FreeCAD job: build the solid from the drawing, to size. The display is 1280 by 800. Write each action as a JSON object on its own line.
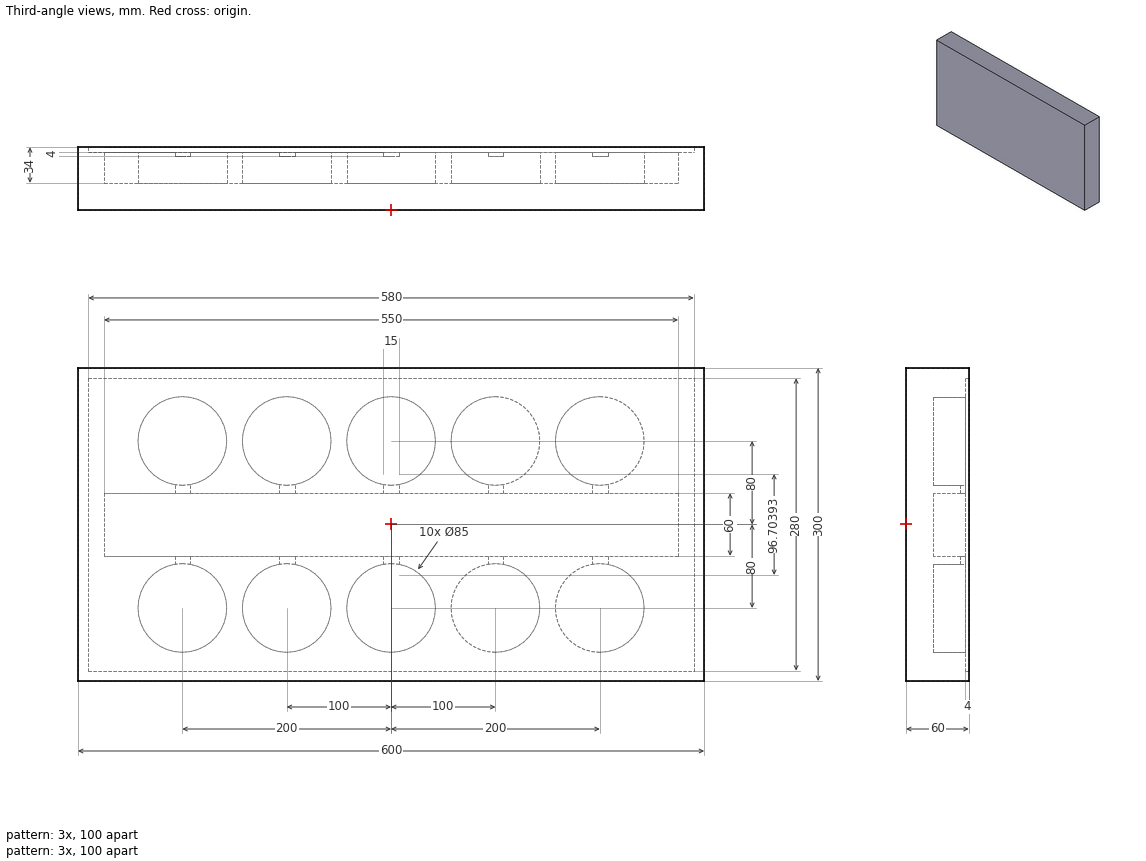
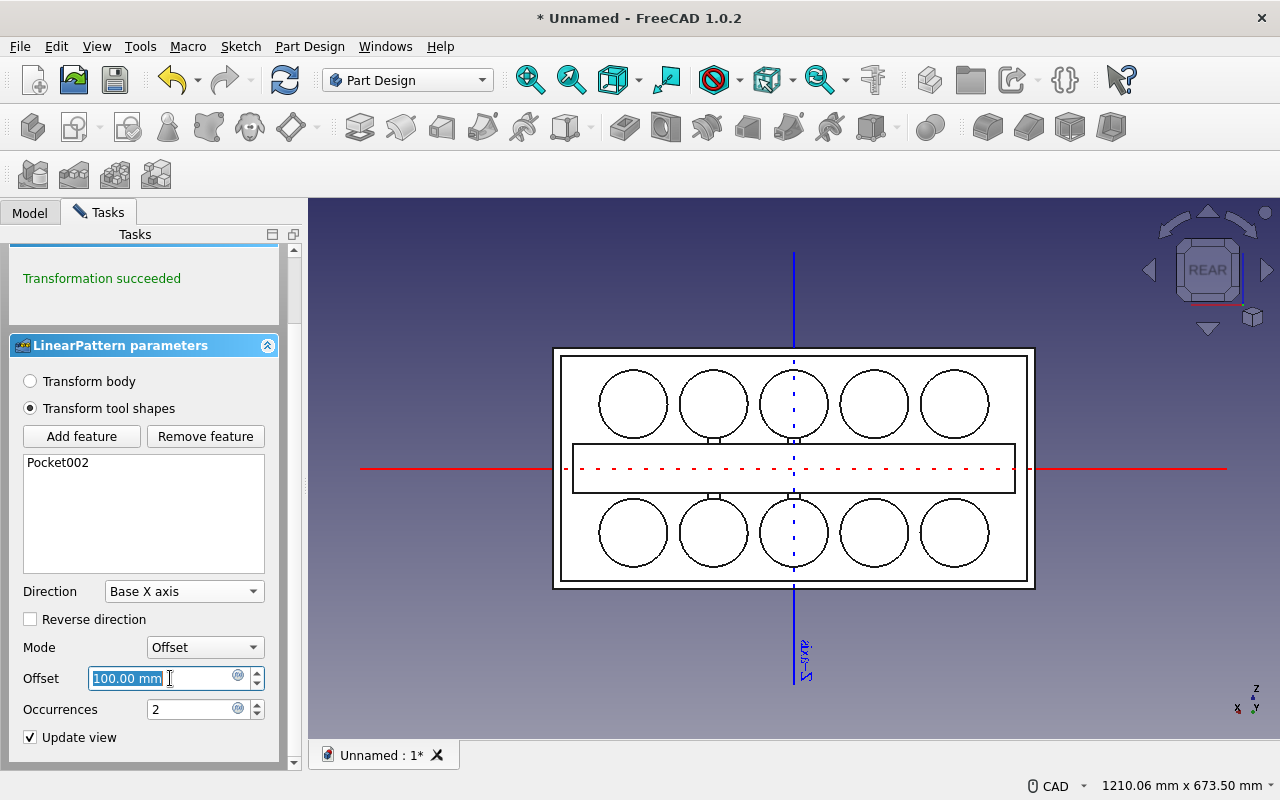
{"action": "type", "text": "100"}
{"action": "key", "text": "Tab"}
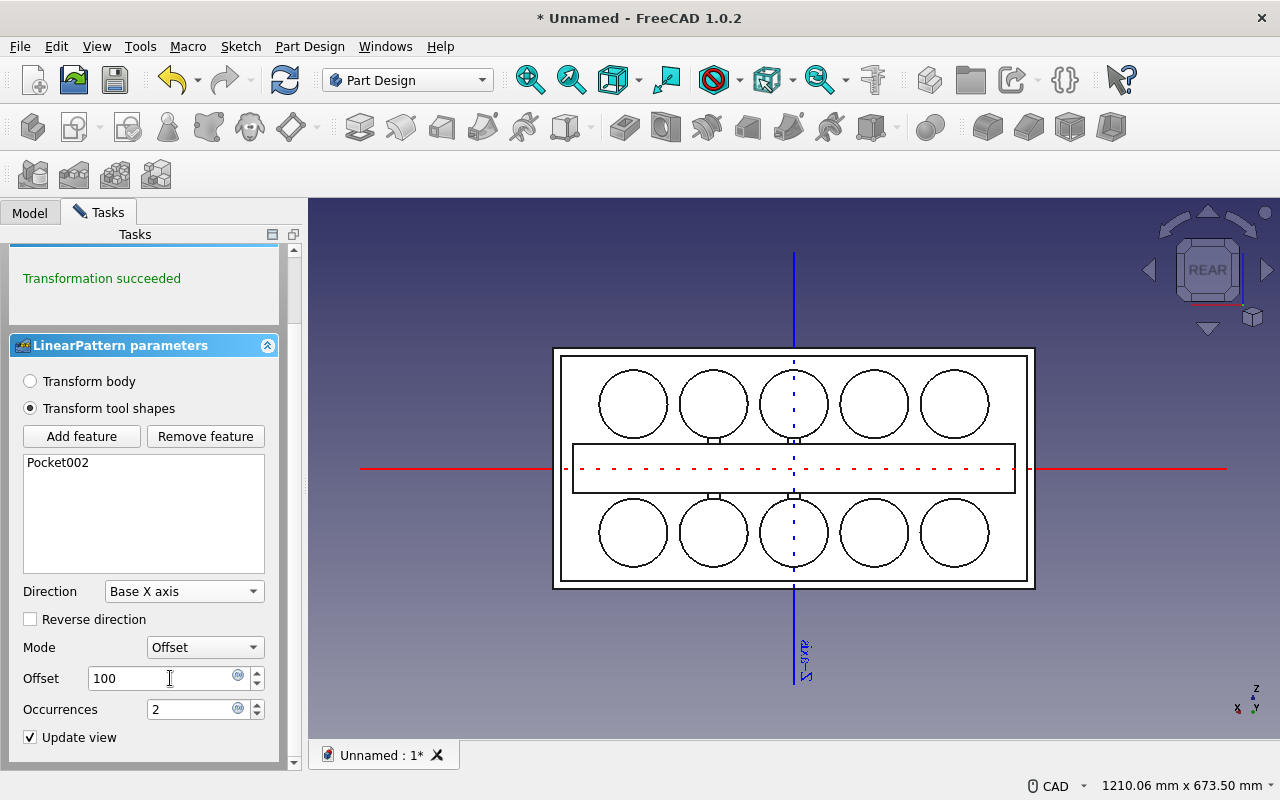
{"action": "triple_click", "coordinate": [199, 710]}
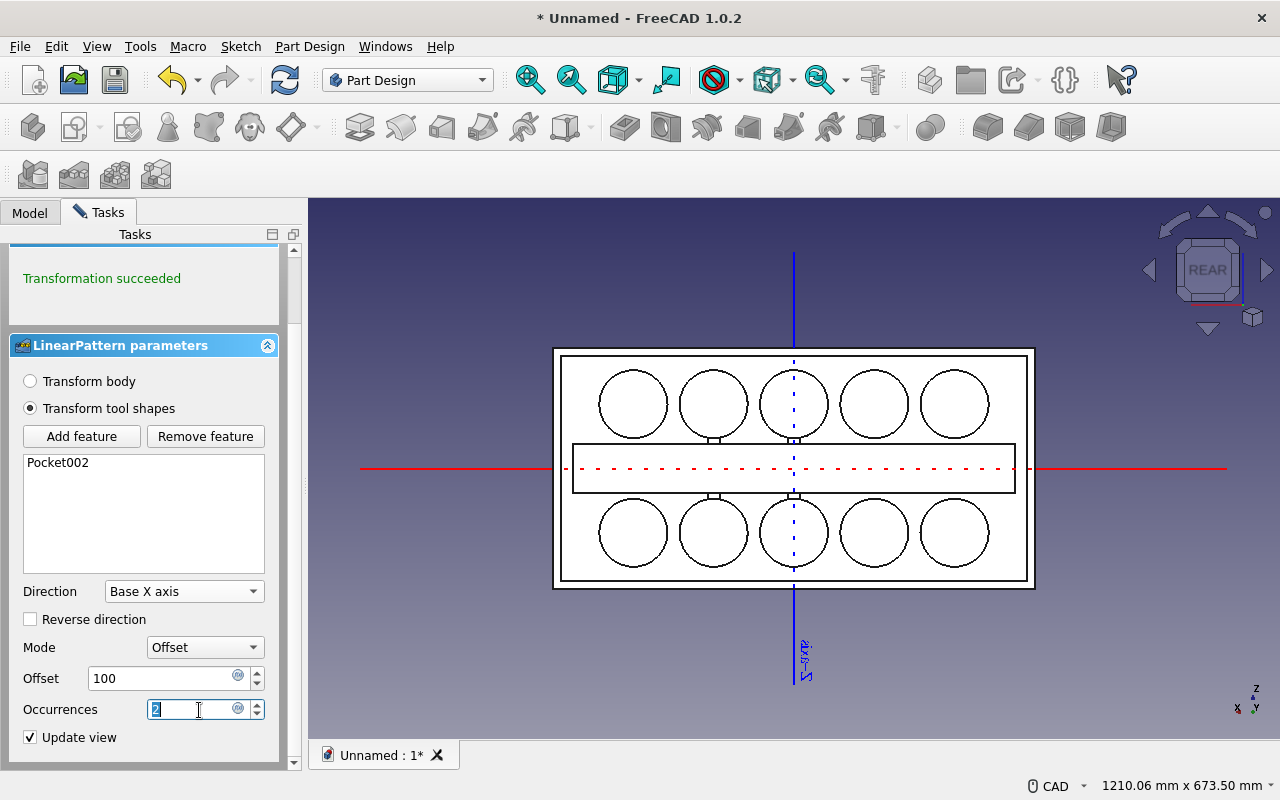
{"action": "type", "text": "3"}
{"action": "key", "text": "Tab"}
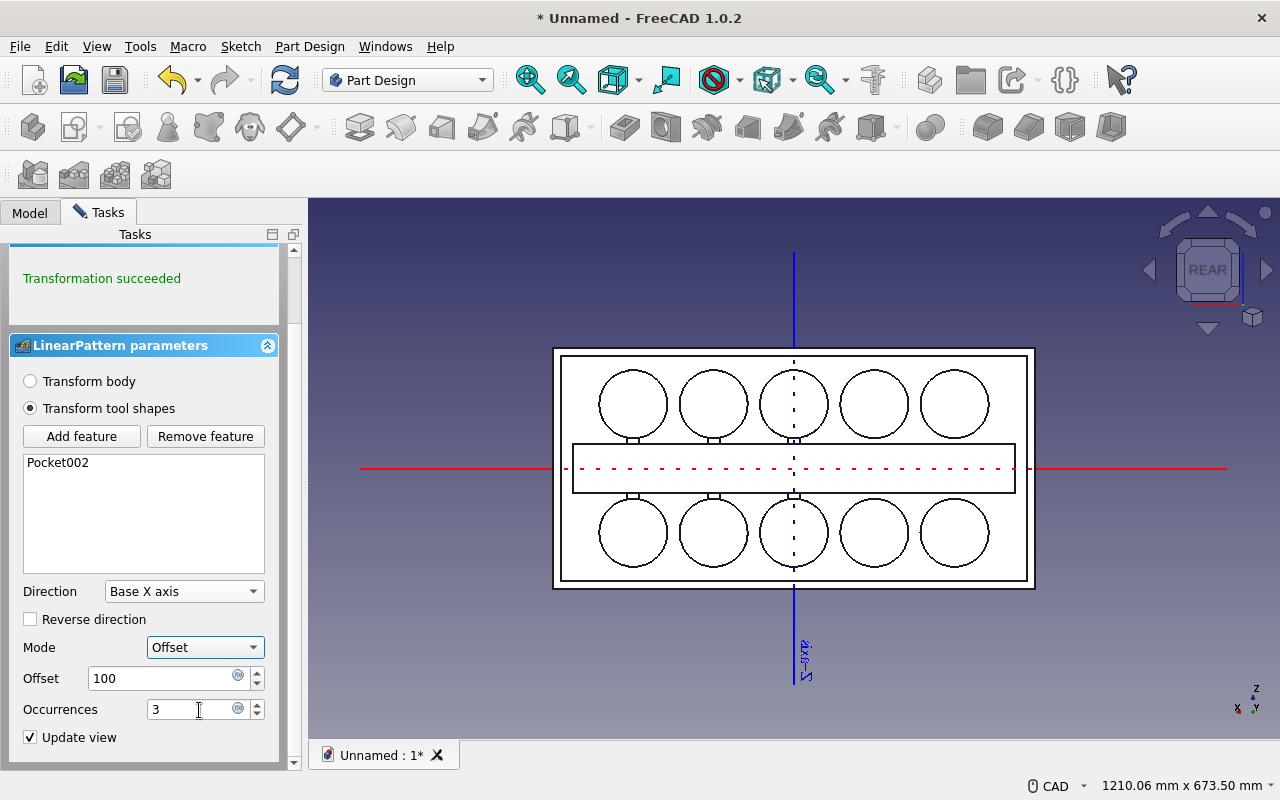
{"action": "left_click", "coordinate": [31, 619]}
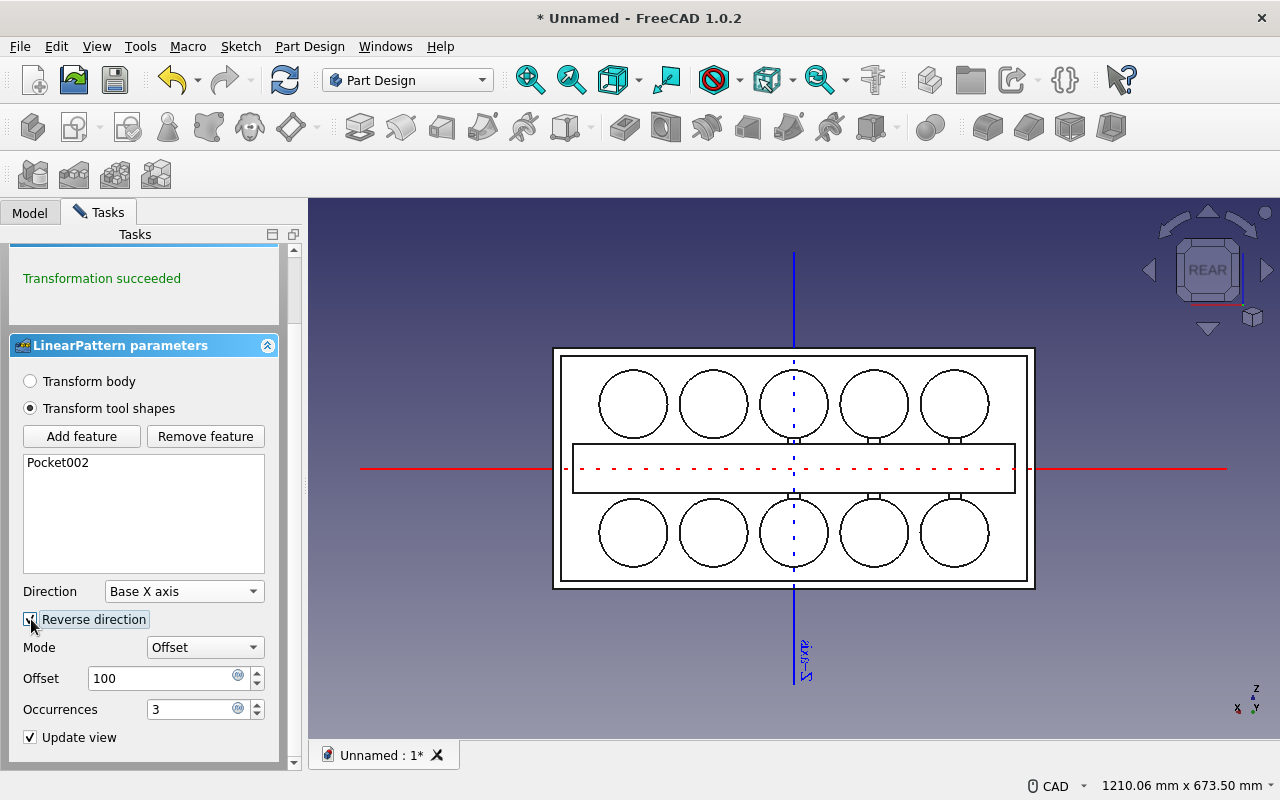
{"action": "scroll", "coordinate": [294, 507], "scroll_direction": "up", "scroll_amount": 3}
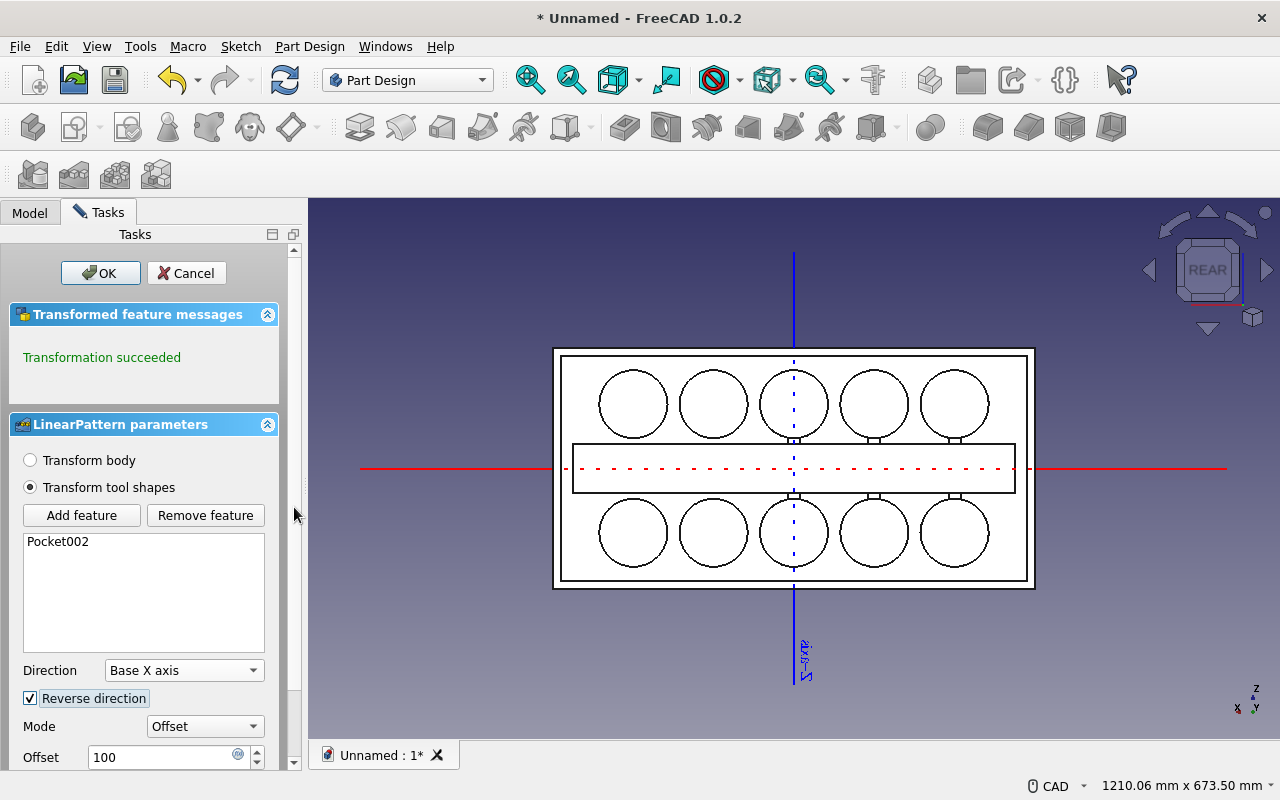
{"action": "left_click", "coordinate": [101, 273]}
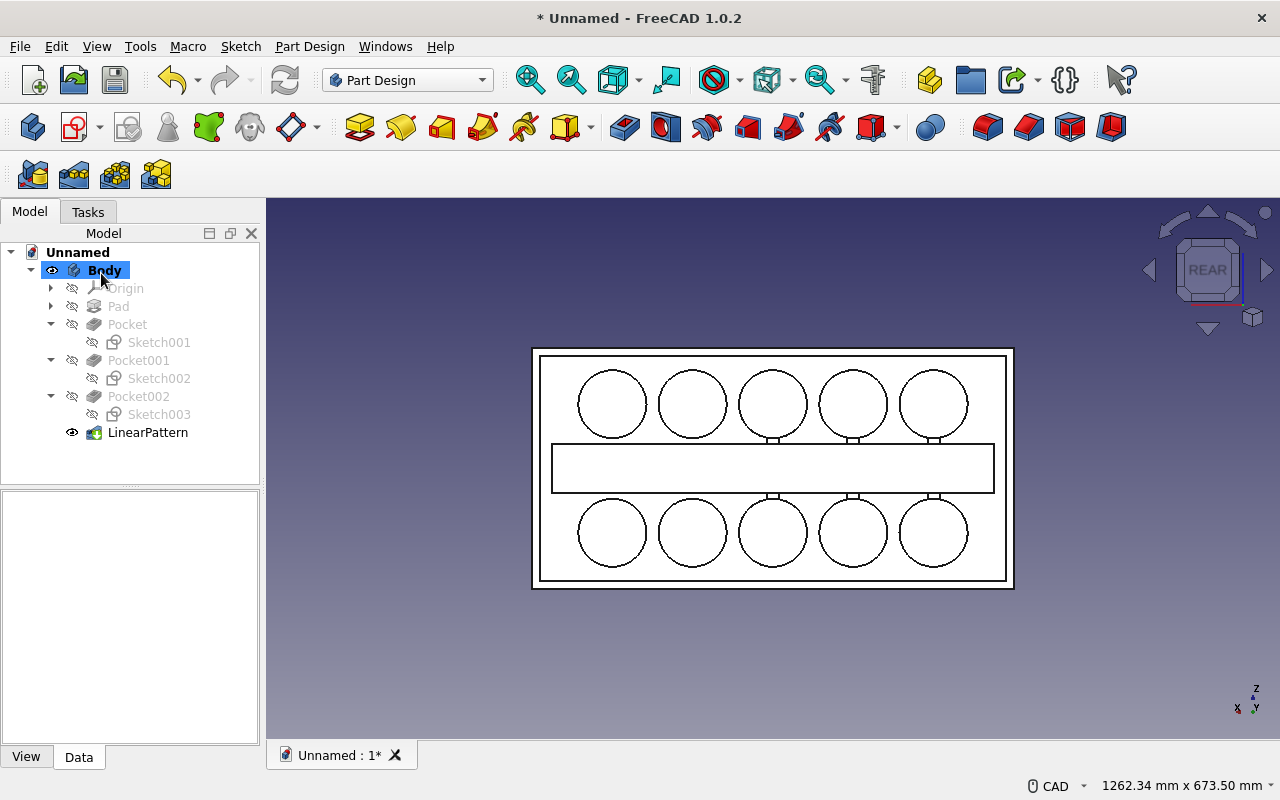
{"action": "left_click", "coordinate": [117, 396]}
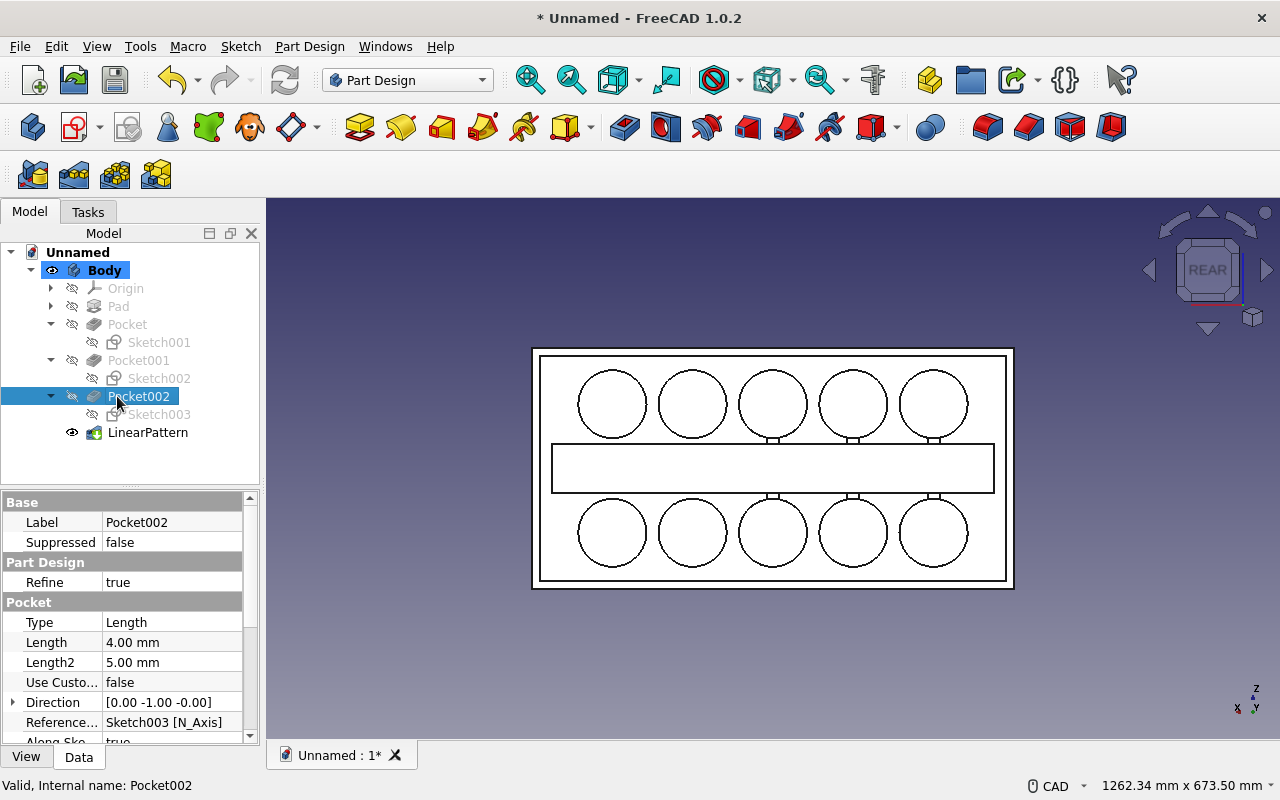
{"action": "left_click", "coordinate": [74, 174]}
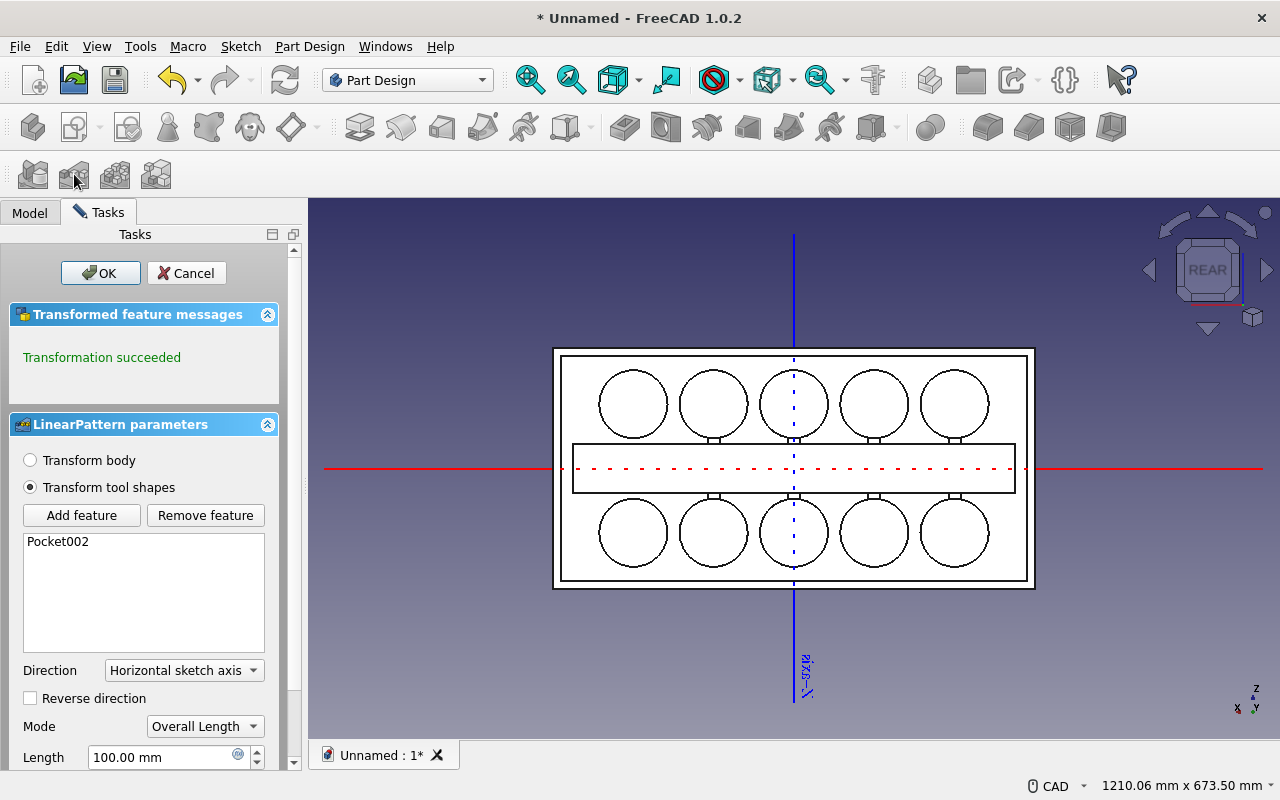
{"action": "left_click", "coordinate": [185, 670]}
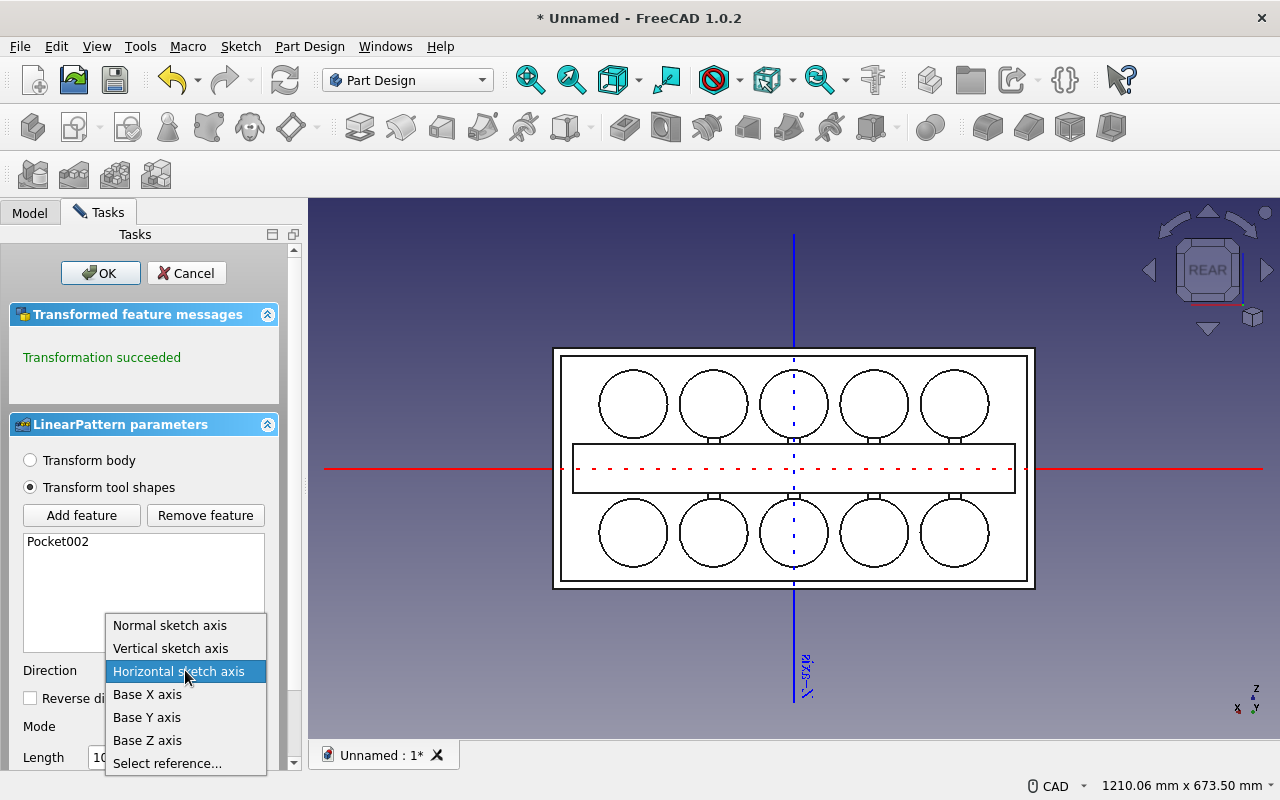
{"action": "left_click", "coordinate": [184, 694]}